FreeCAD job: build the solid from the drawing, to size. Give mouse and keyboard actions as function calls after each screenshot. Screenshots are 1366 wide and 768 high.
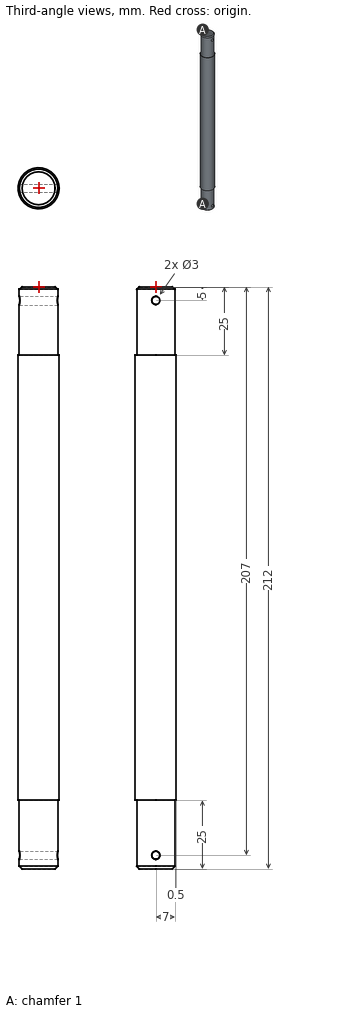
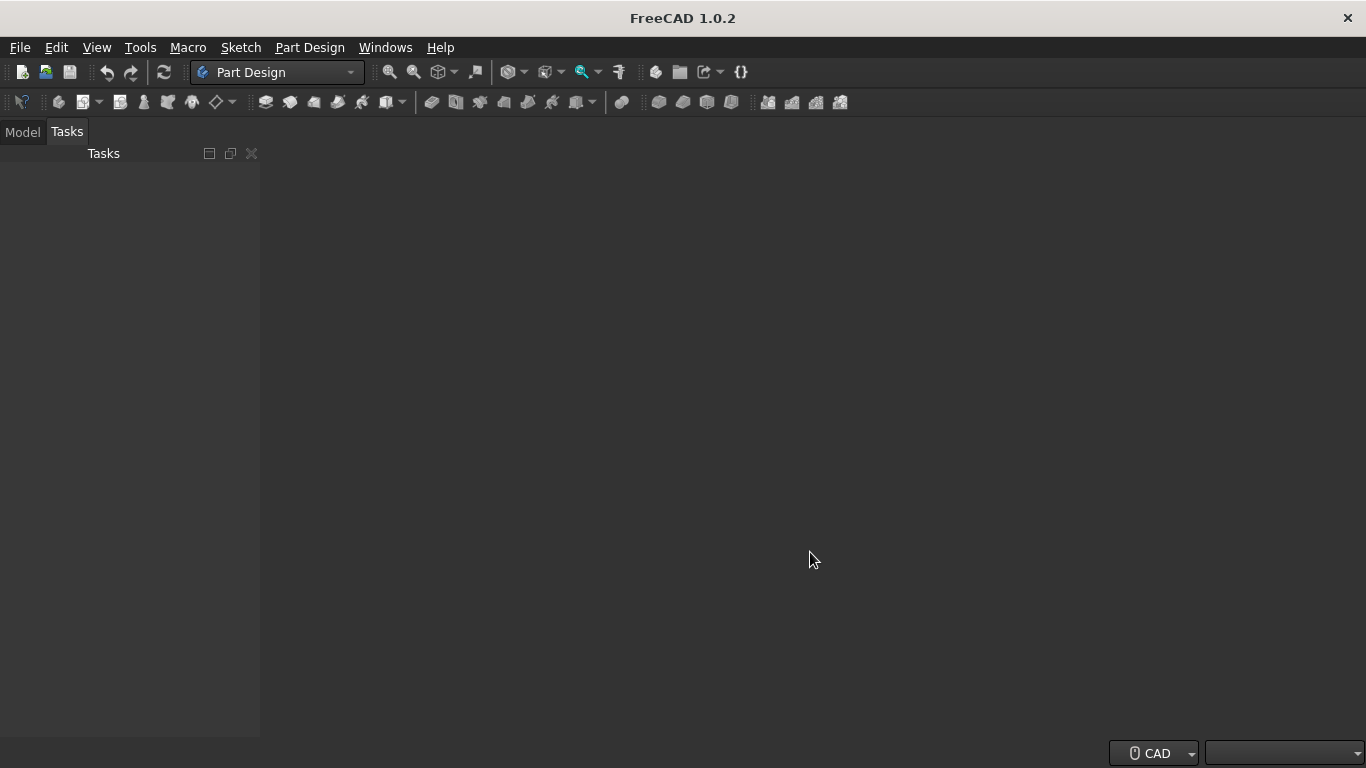
key(ctrl+n)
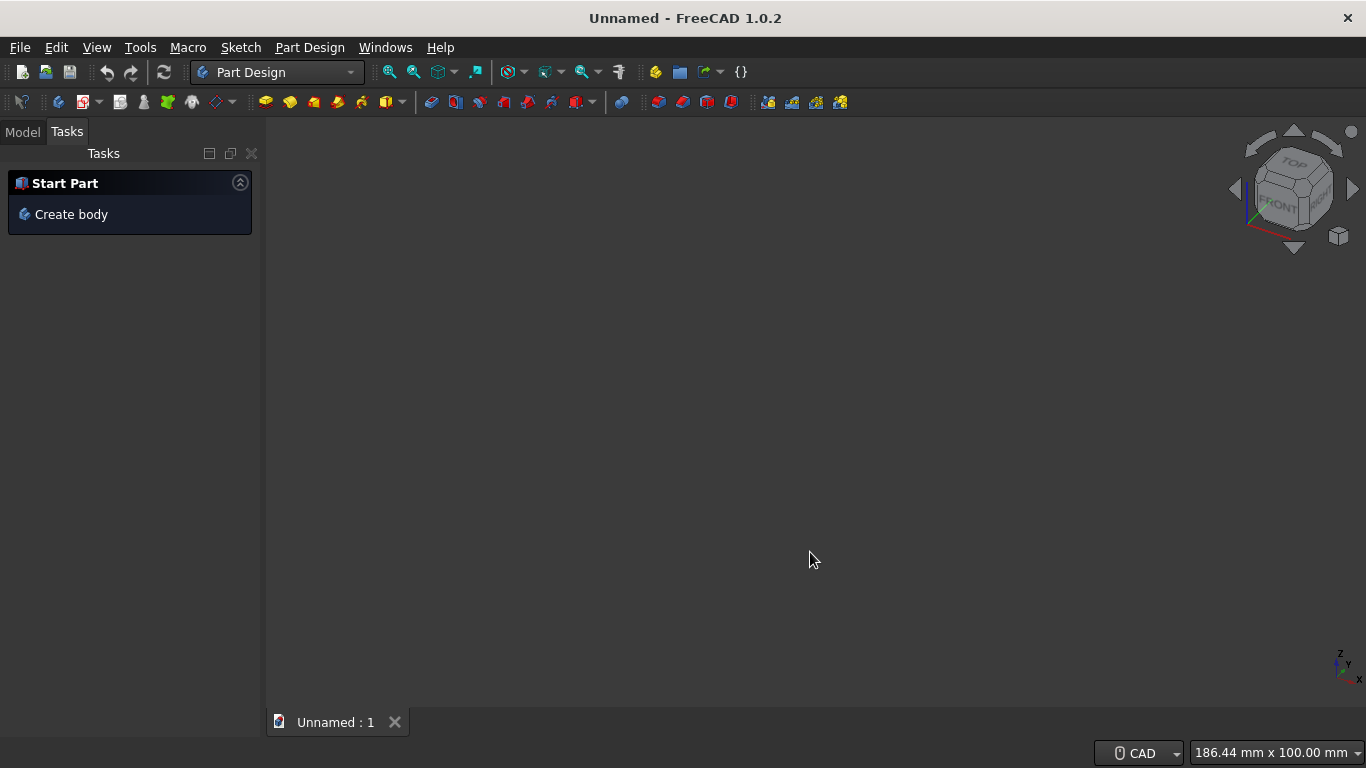
click(84, 102)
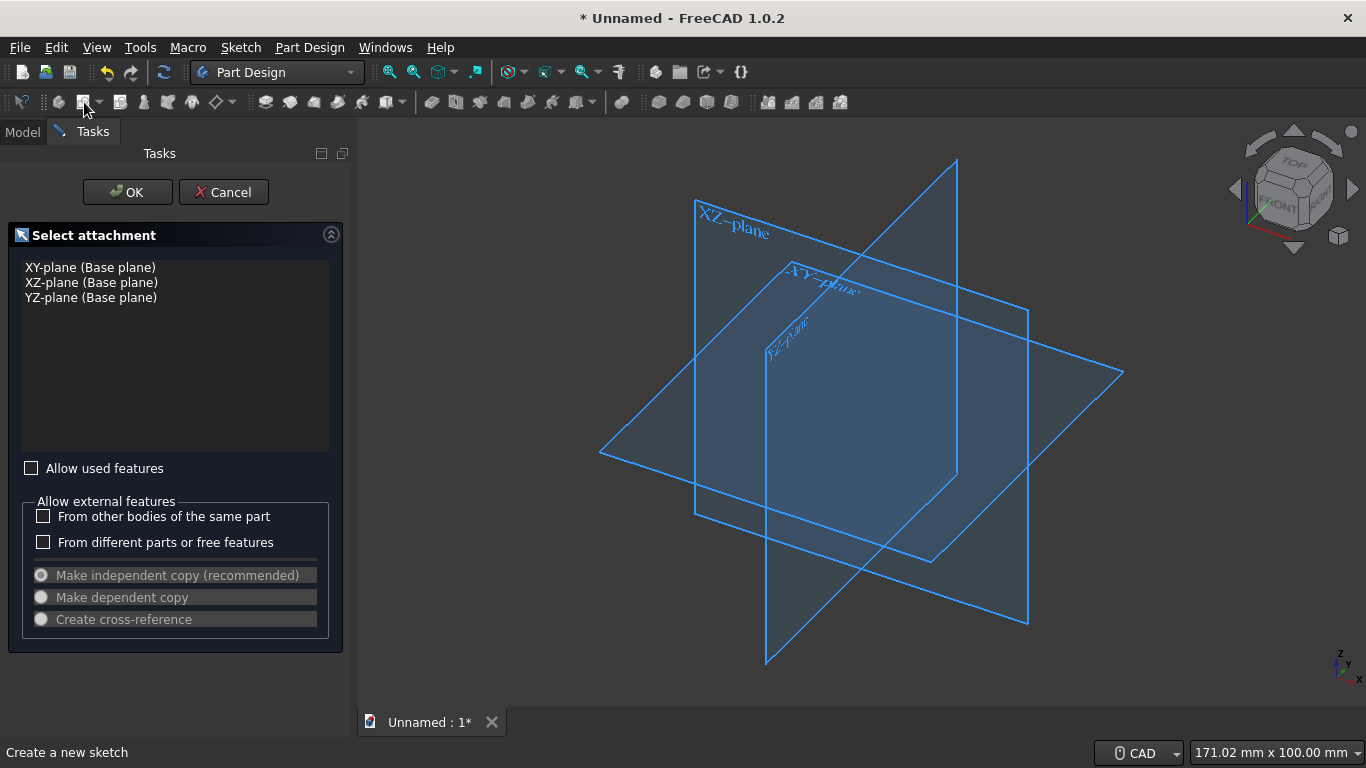
click(82, 298)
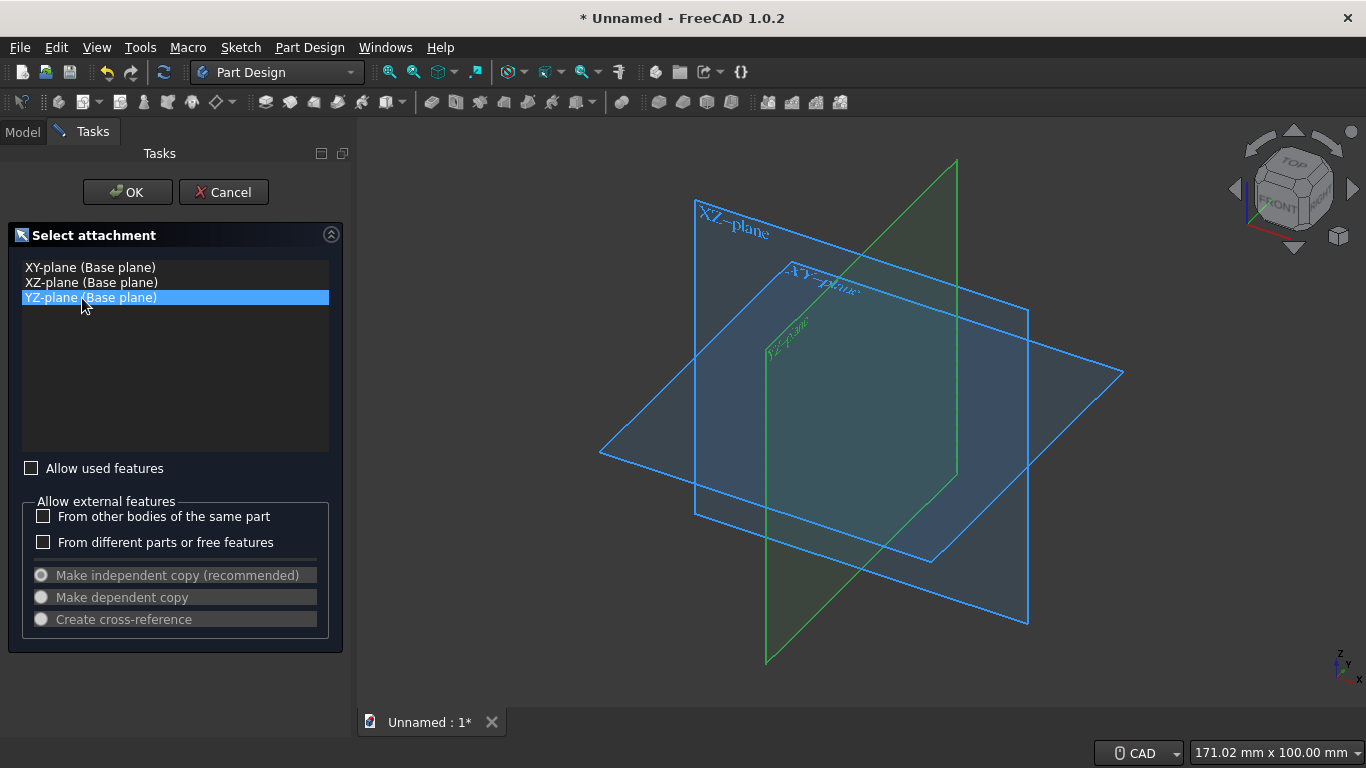
click(128, 192)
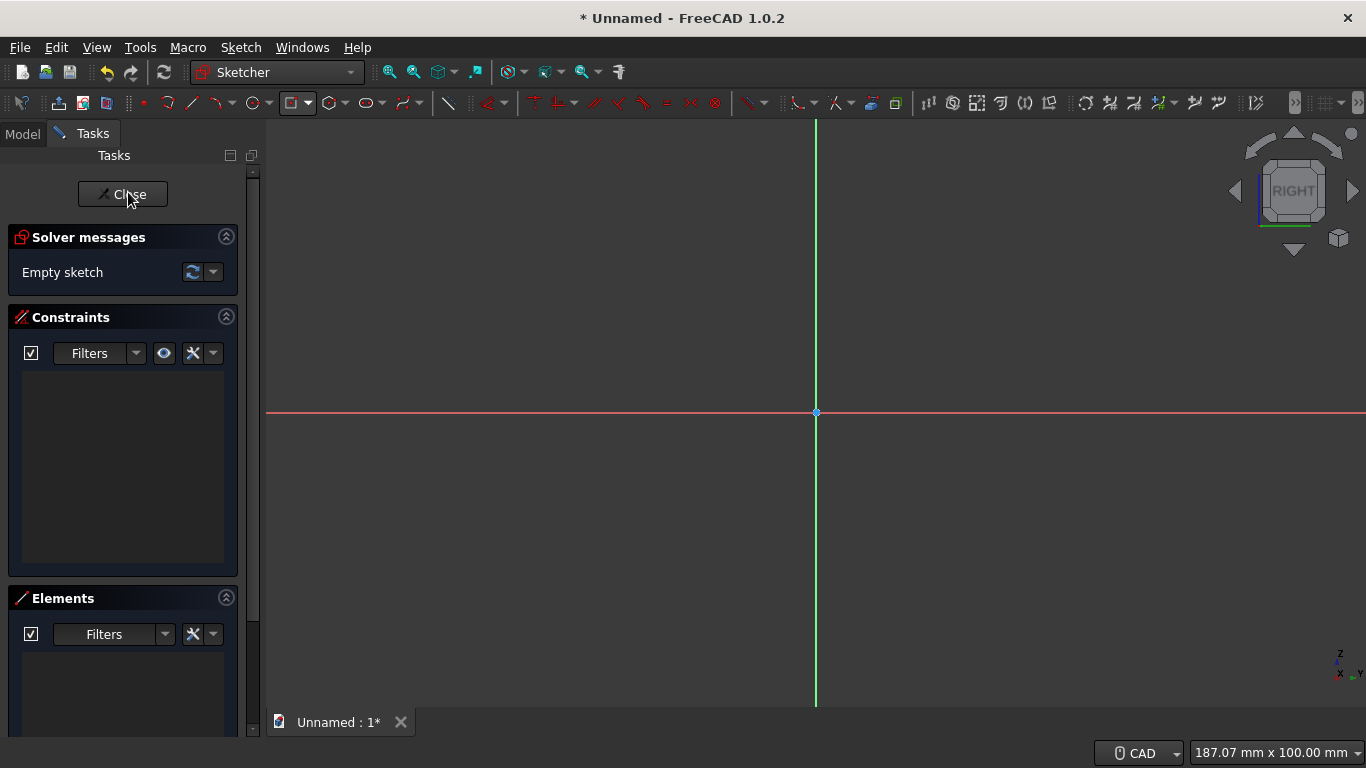
scroll(708, 147, down, 6)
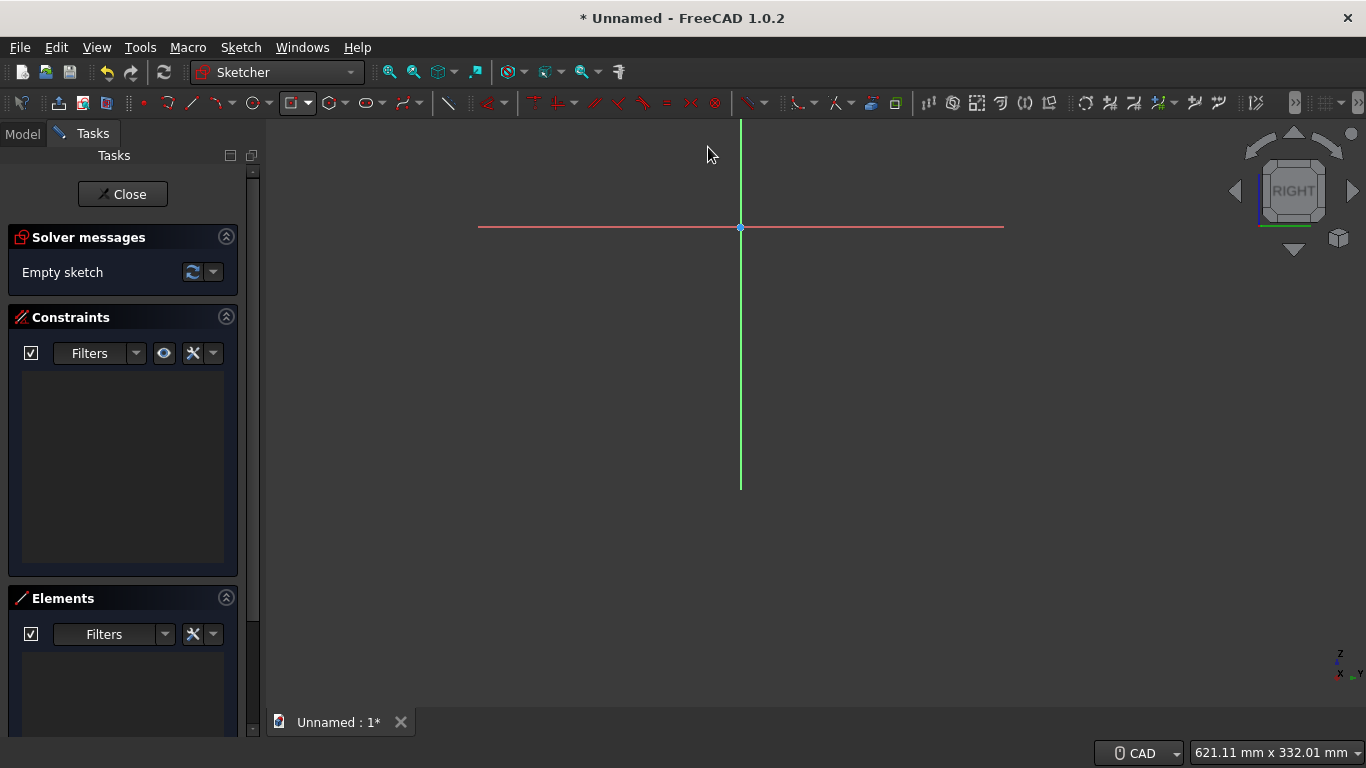
click(168, 104)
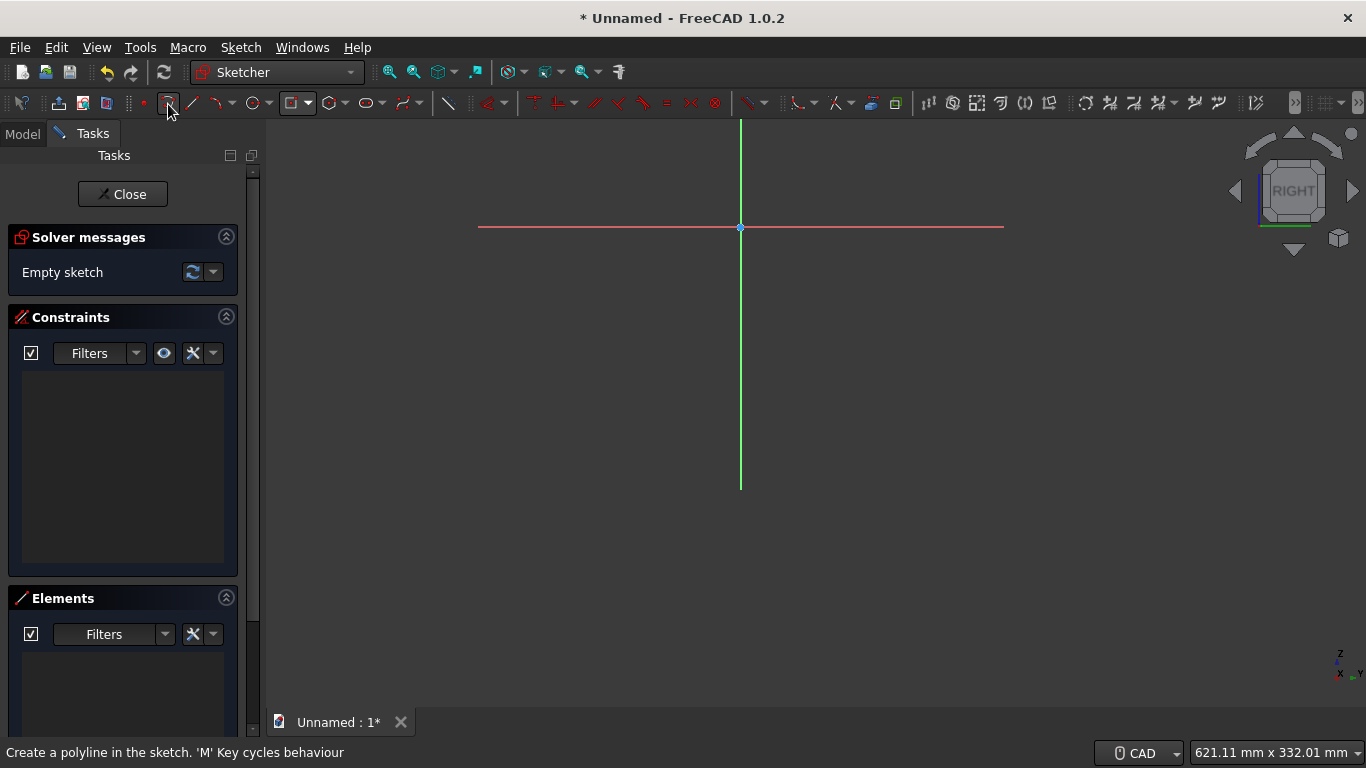
click(741, 227)
click(750, 603)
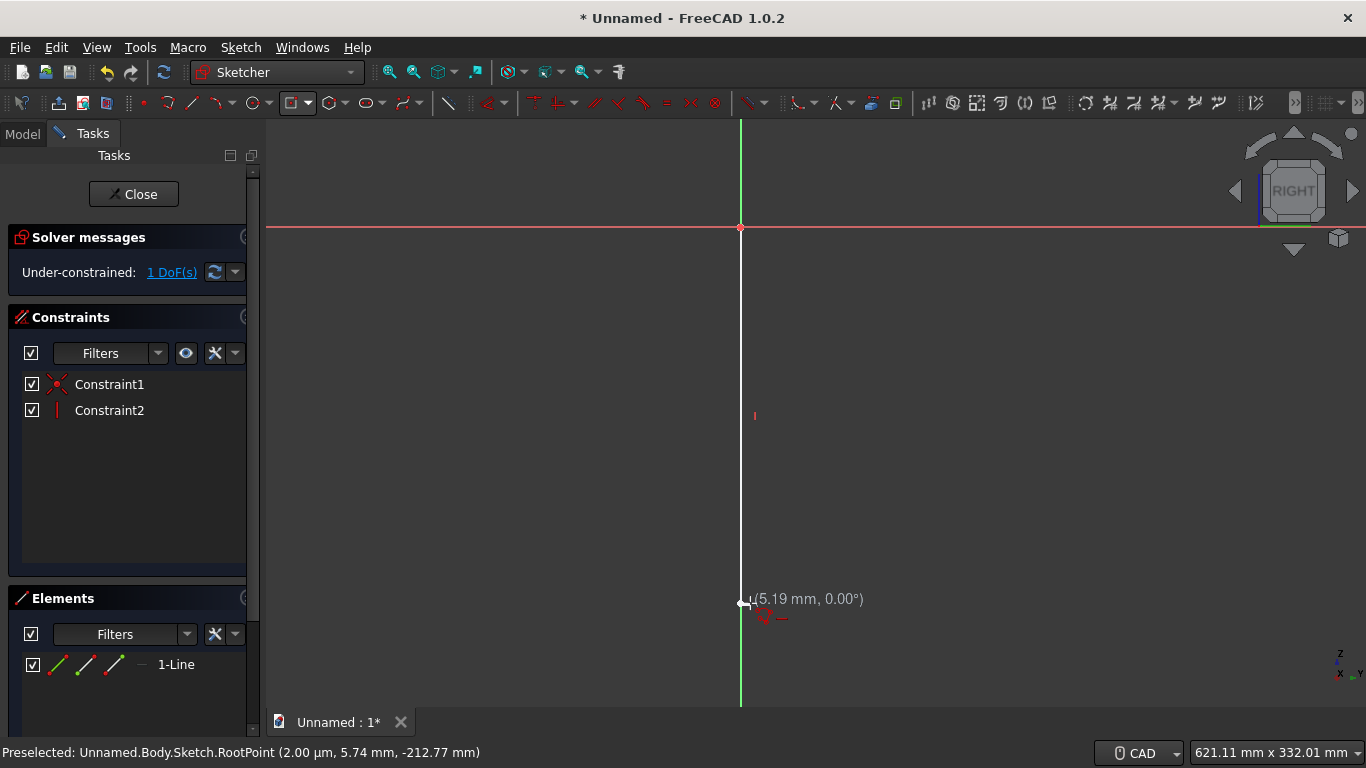
scroll(753, 603, up, 2)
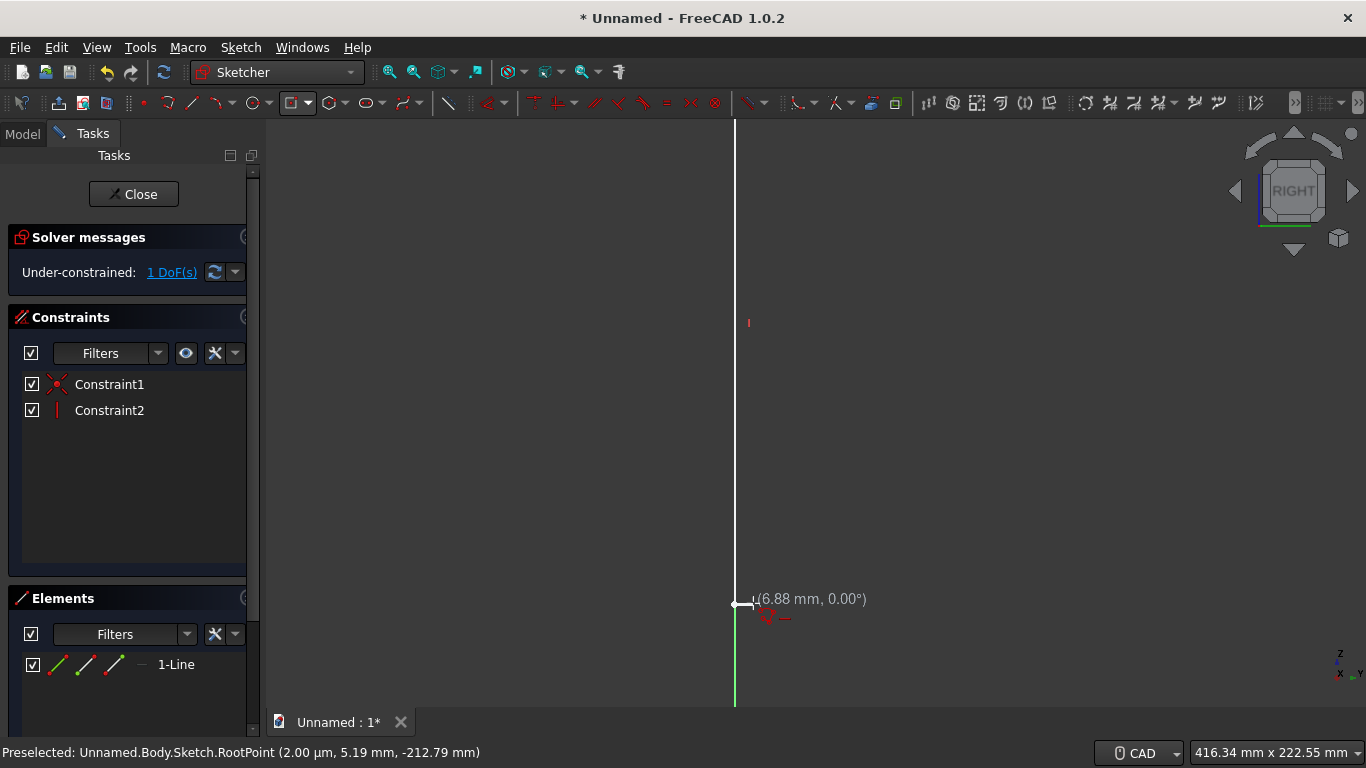
click(753, 603)
click(753, 536)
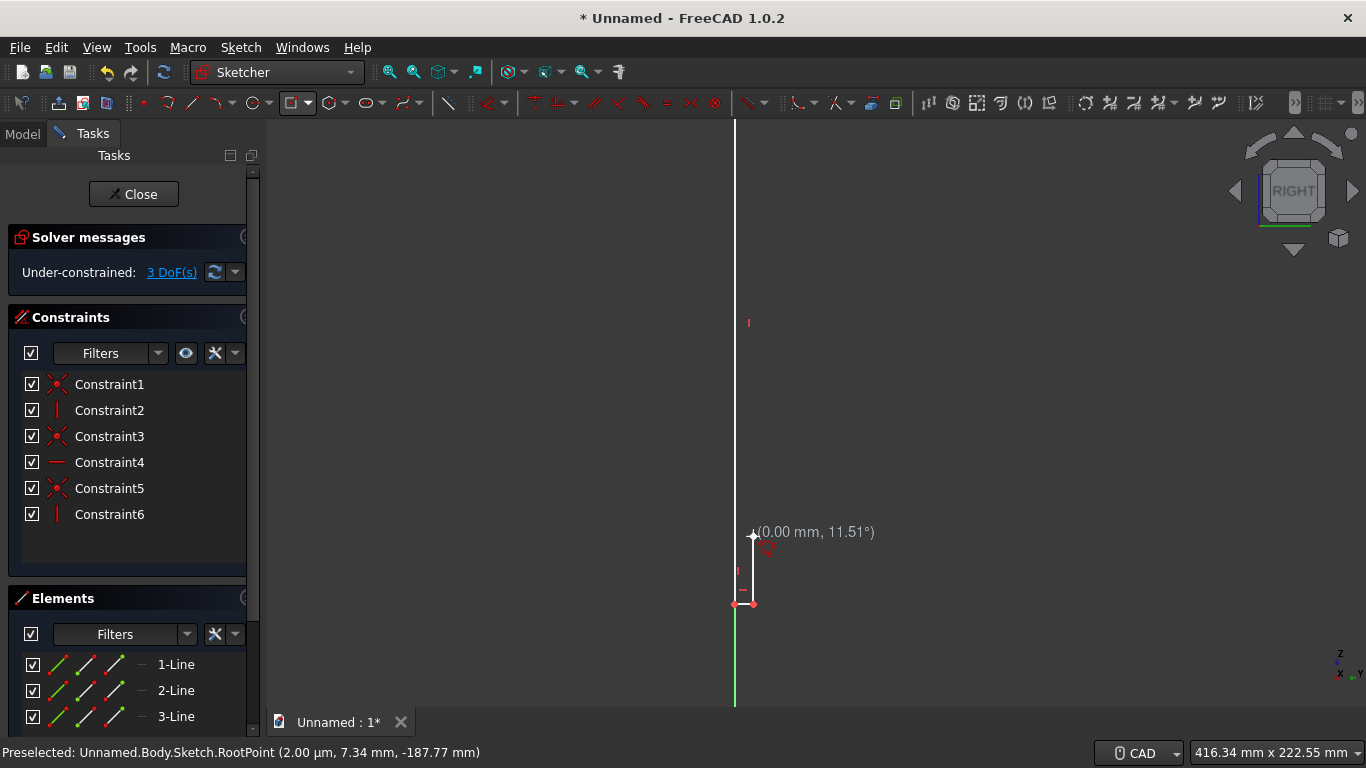
scroll(754, 536, up, 13)